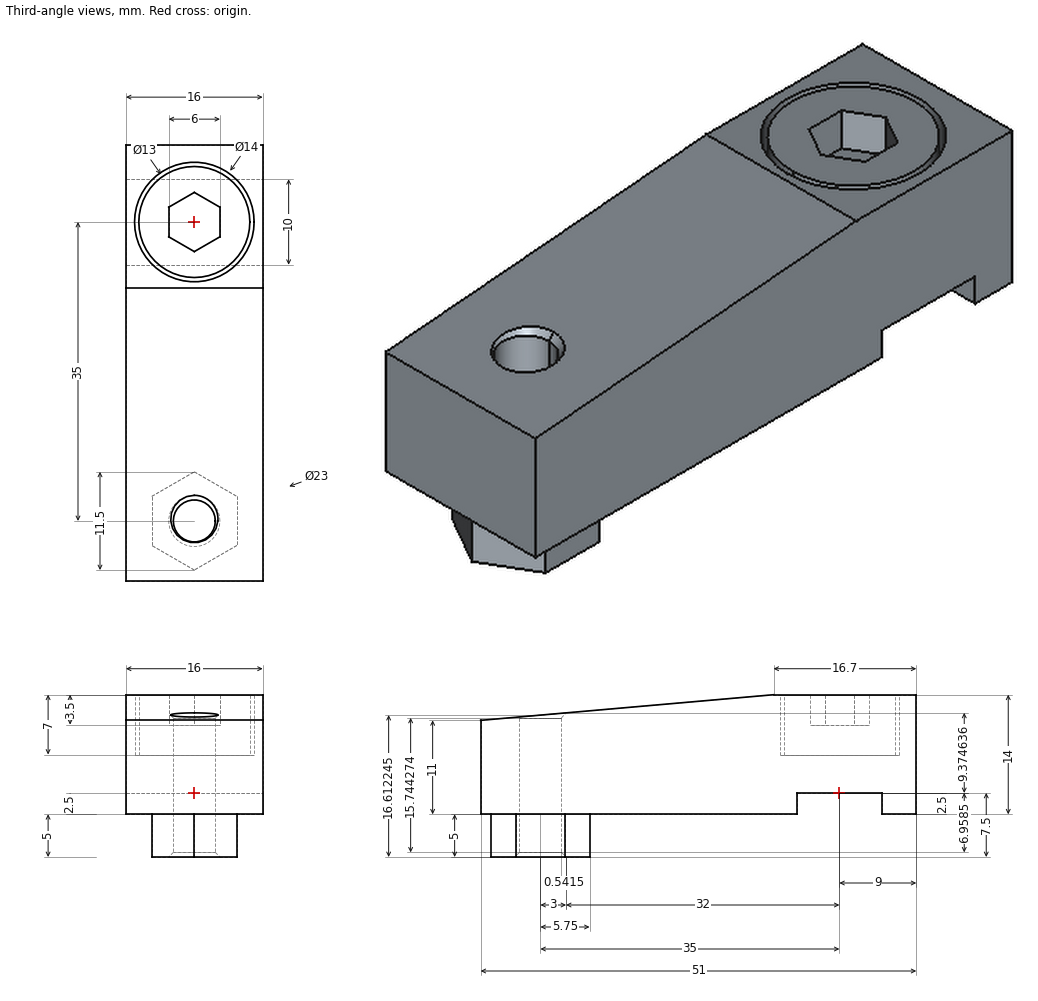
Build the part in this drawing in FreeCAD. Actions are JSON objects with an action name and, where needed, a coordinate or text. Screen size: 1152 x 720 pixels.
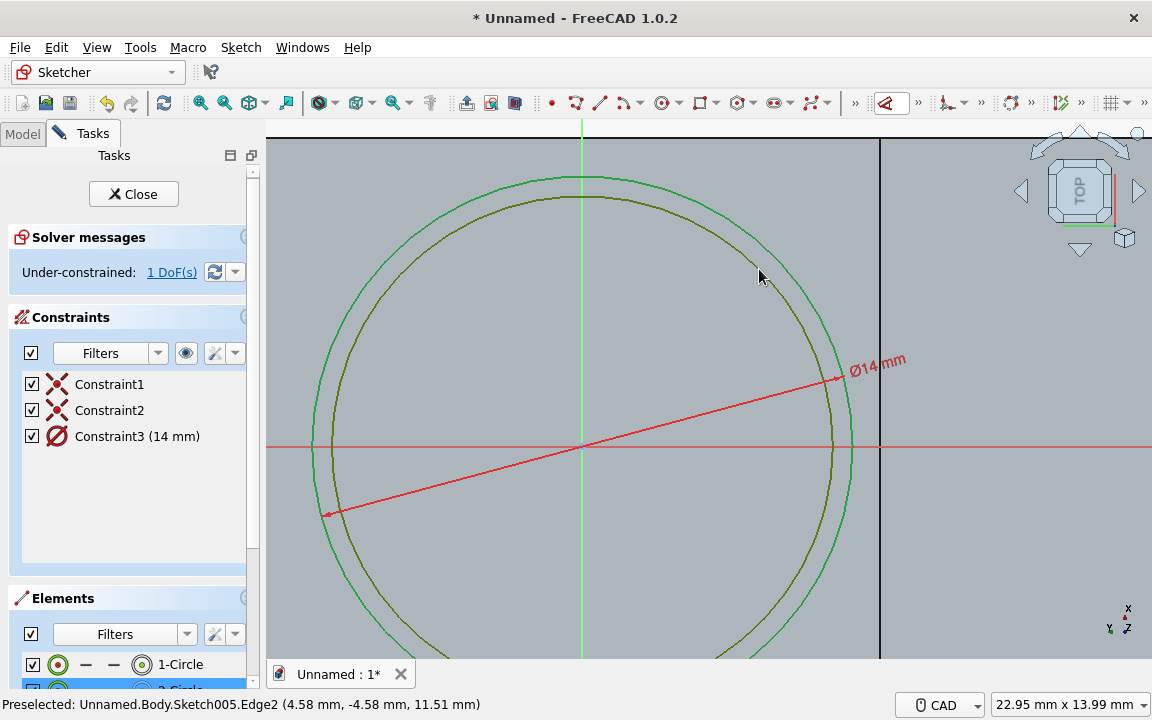
{"action": "key", "text": "k o"}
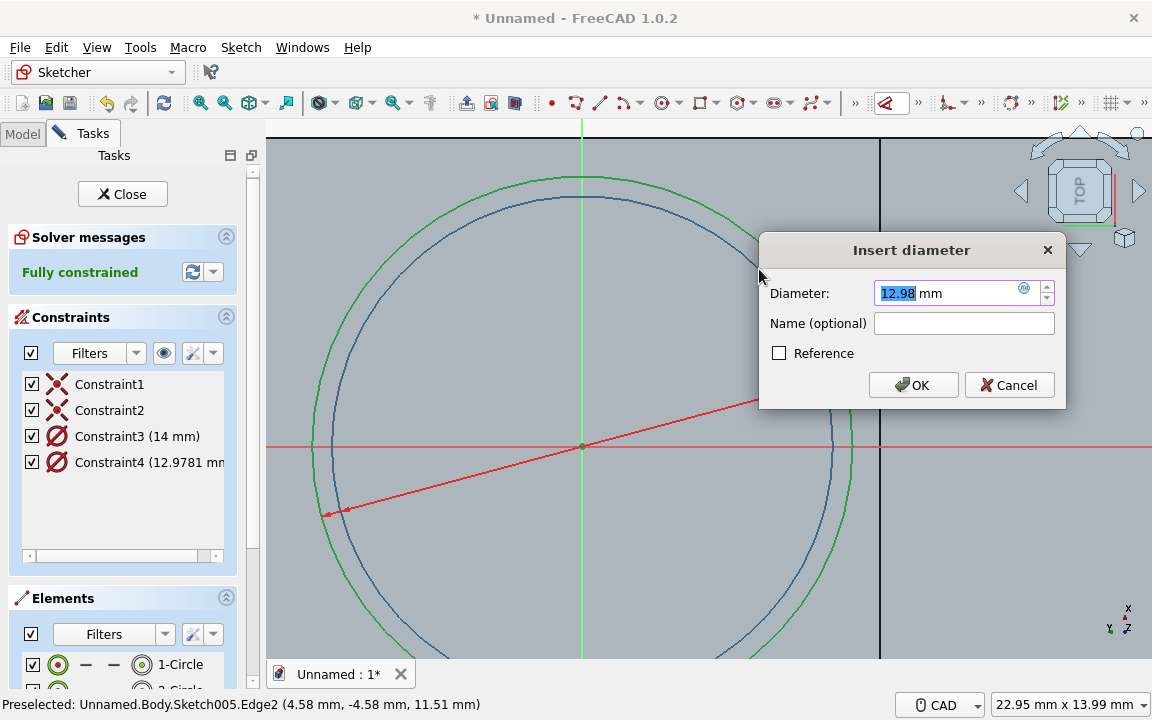
{"action": "type", "text": "13"}
{"action": "key", "text": "Return"}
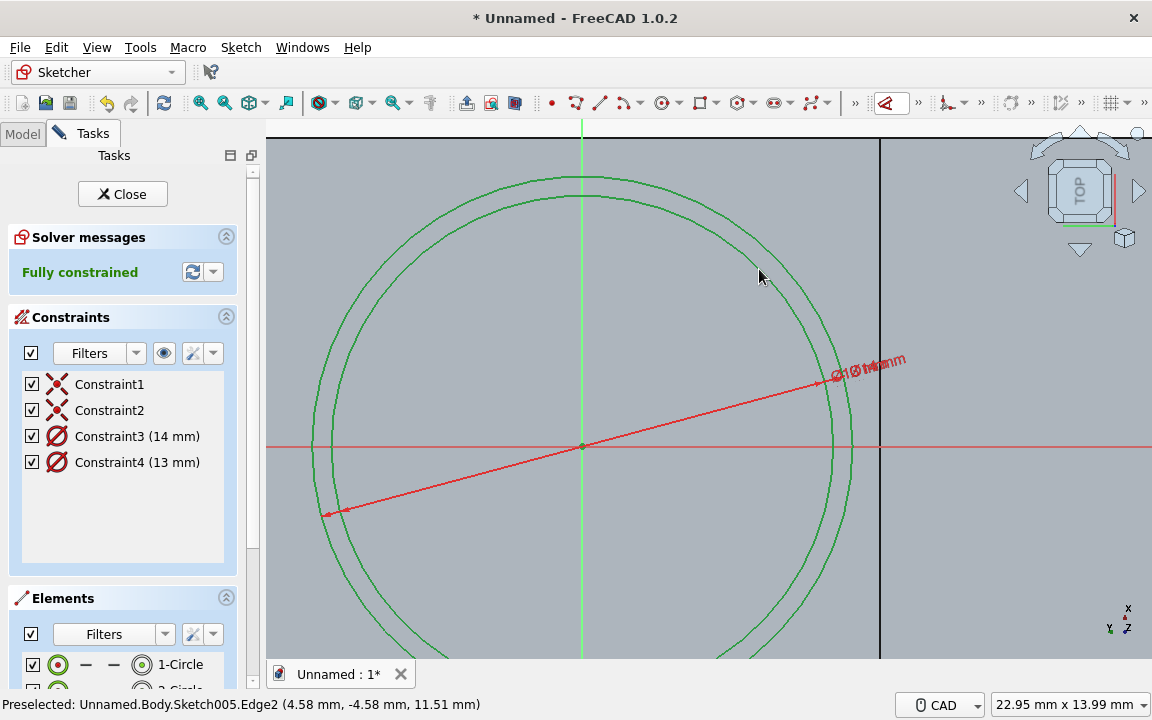
{"action": "left_click", "coordinate": [123, 194]}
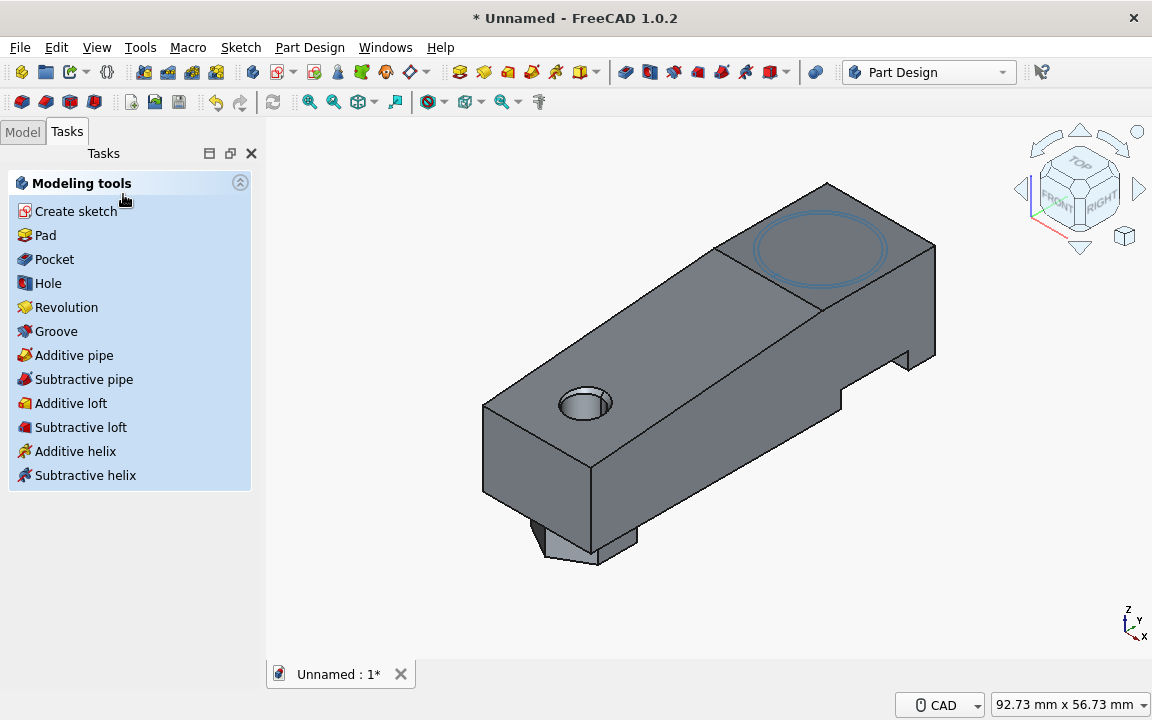
{"action": "left_click", "coordinate": [626, 72]}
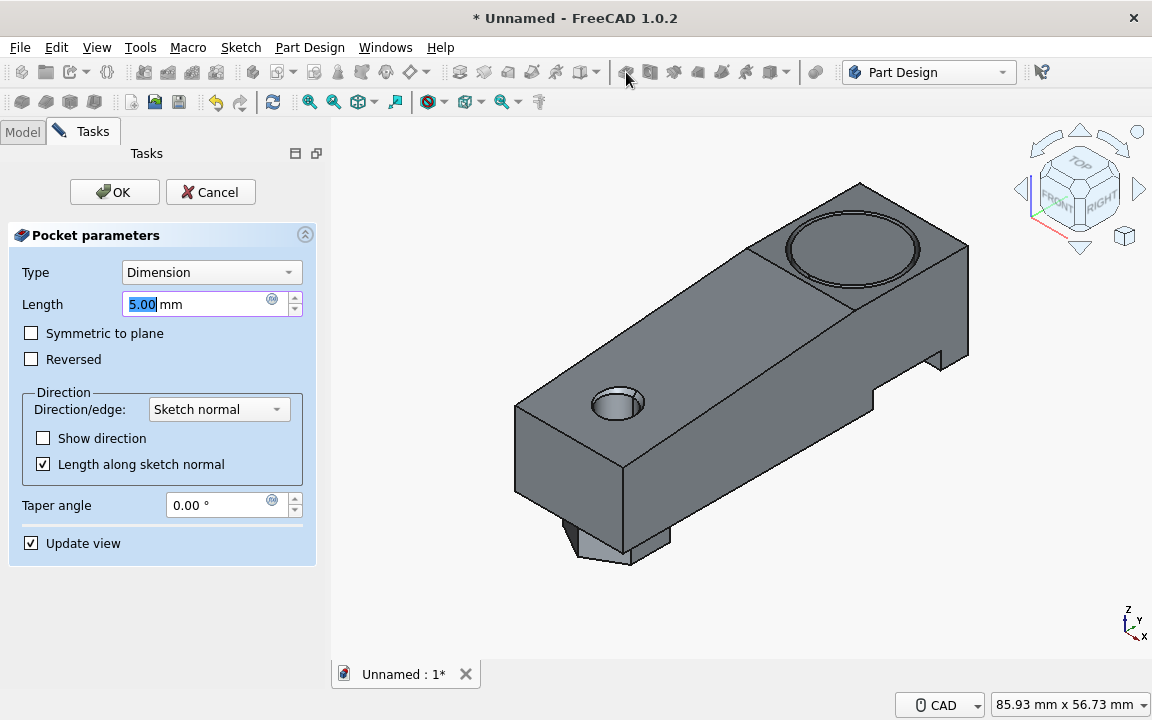
{"action": "type", "text": "7"}
{"action": "key", "text": "Tab"}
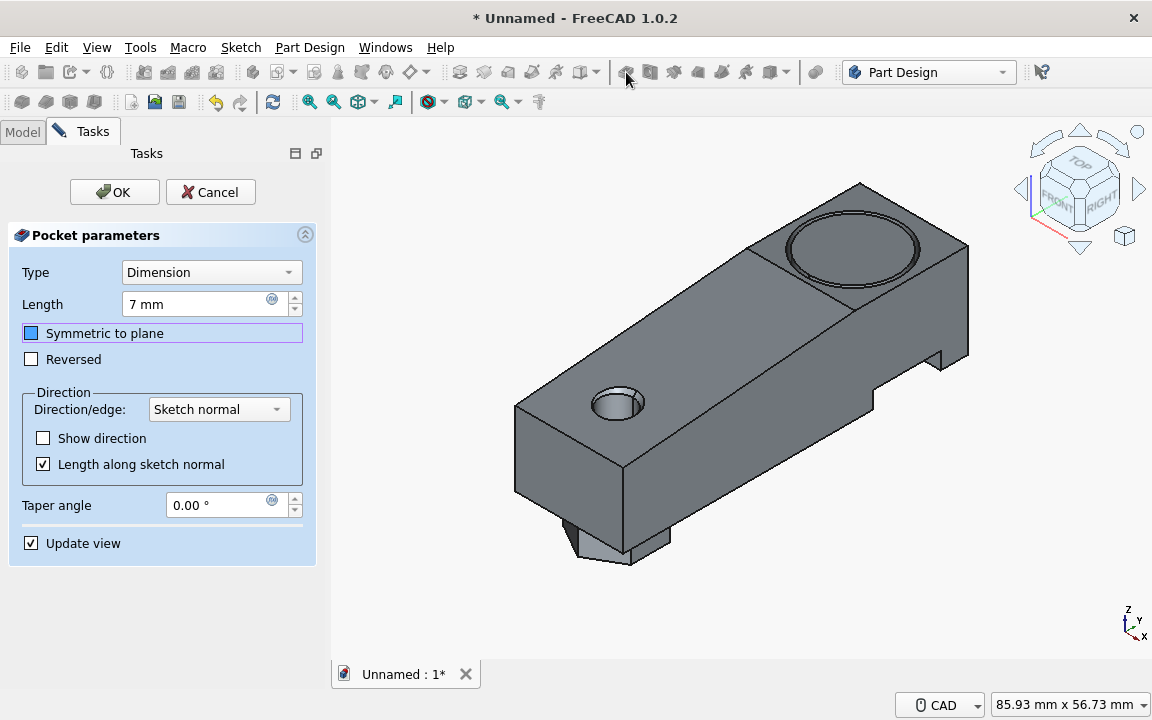
{"action": "left_click", "coordinate": [115, 192]}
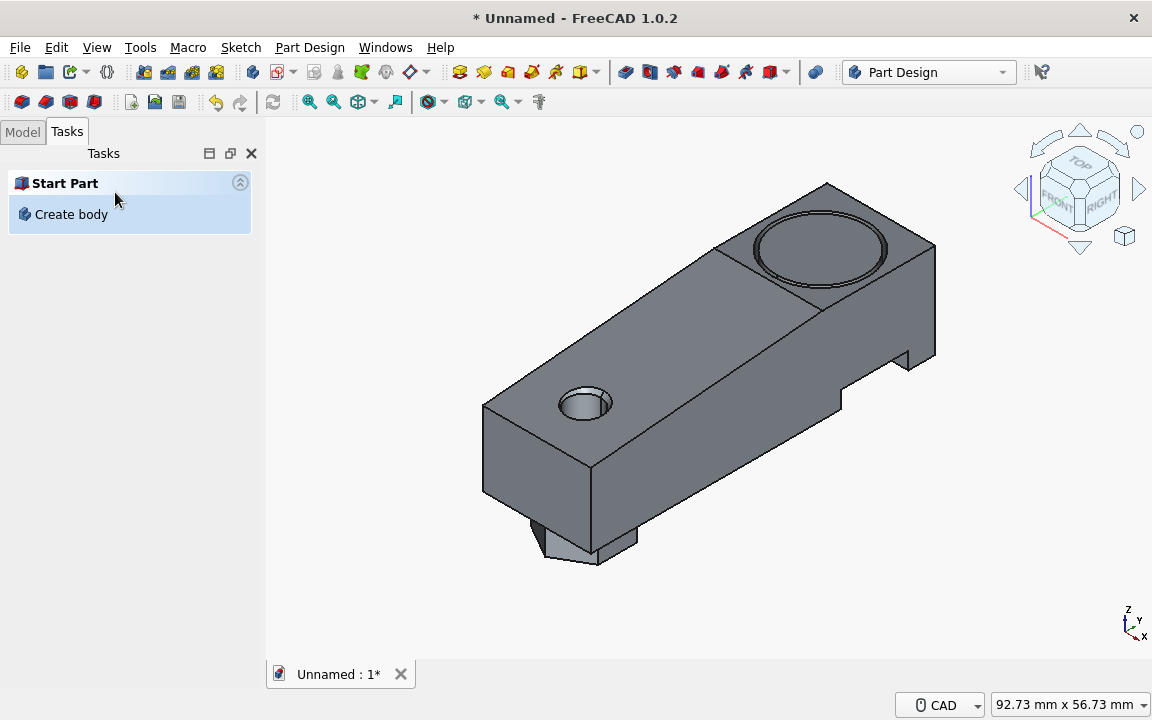
{"action": "left_click", "coordinate": [820, 249]}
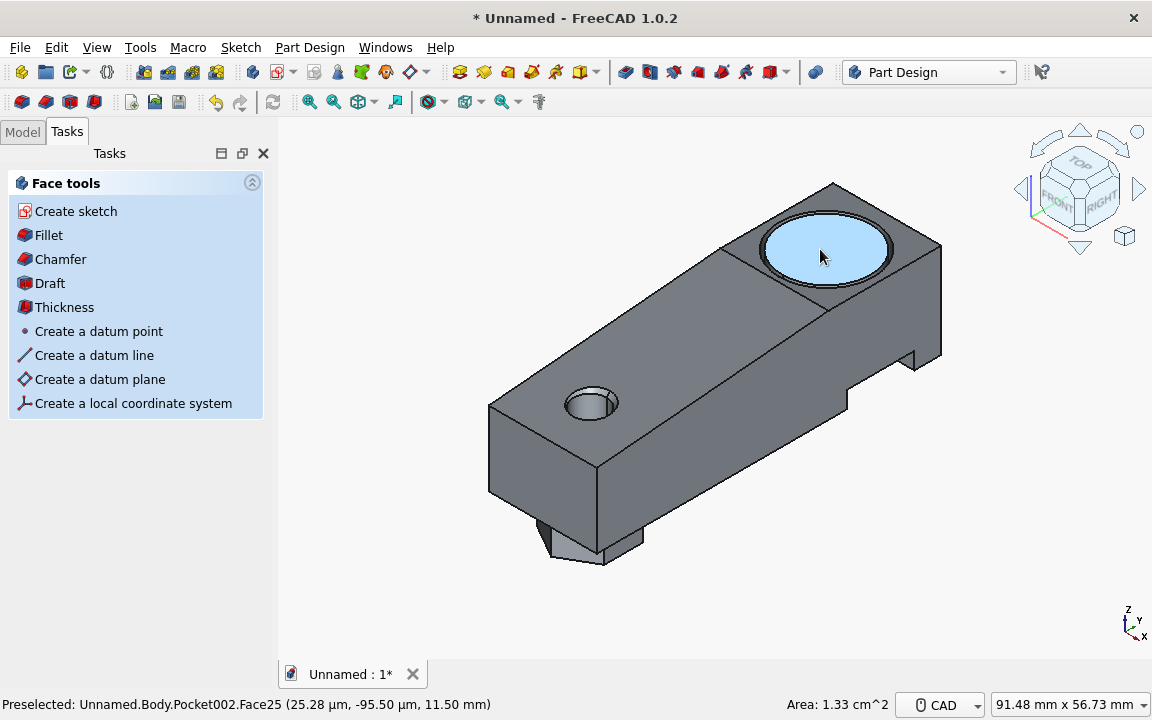
{"action": "left_click", "coordinate": [278, 72]}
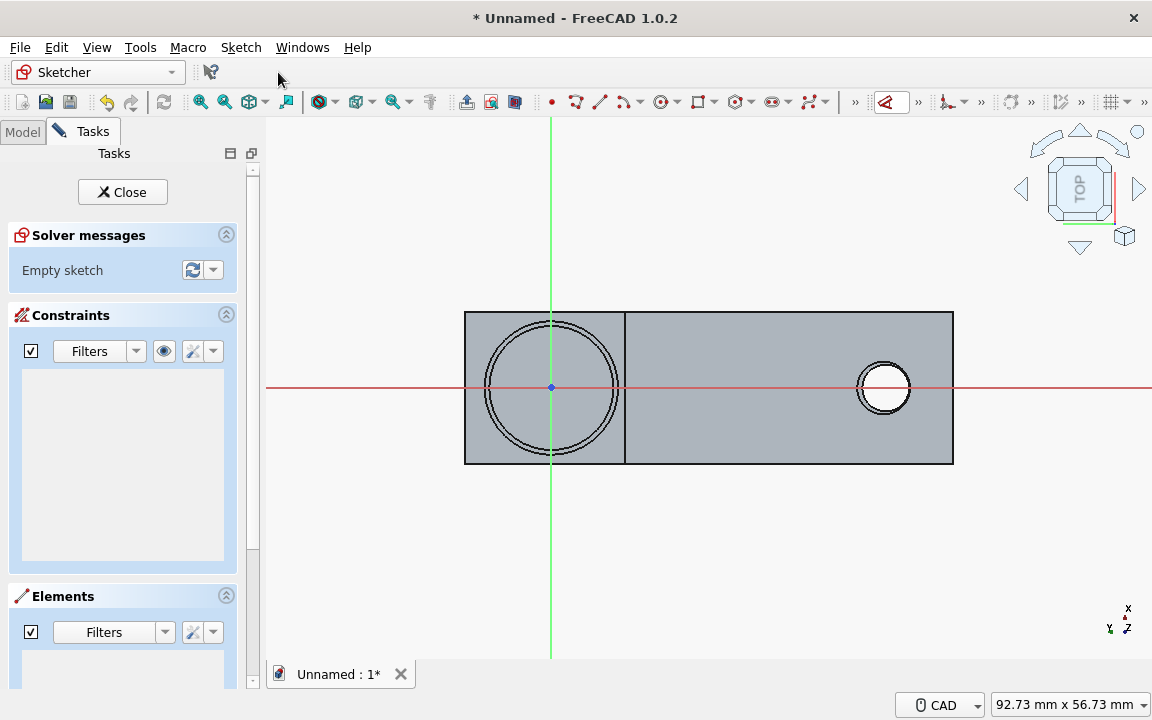
{"action": "scroll", "coordinate": [534, 388], "scroll_direction": "up", "scroll_amount": 9}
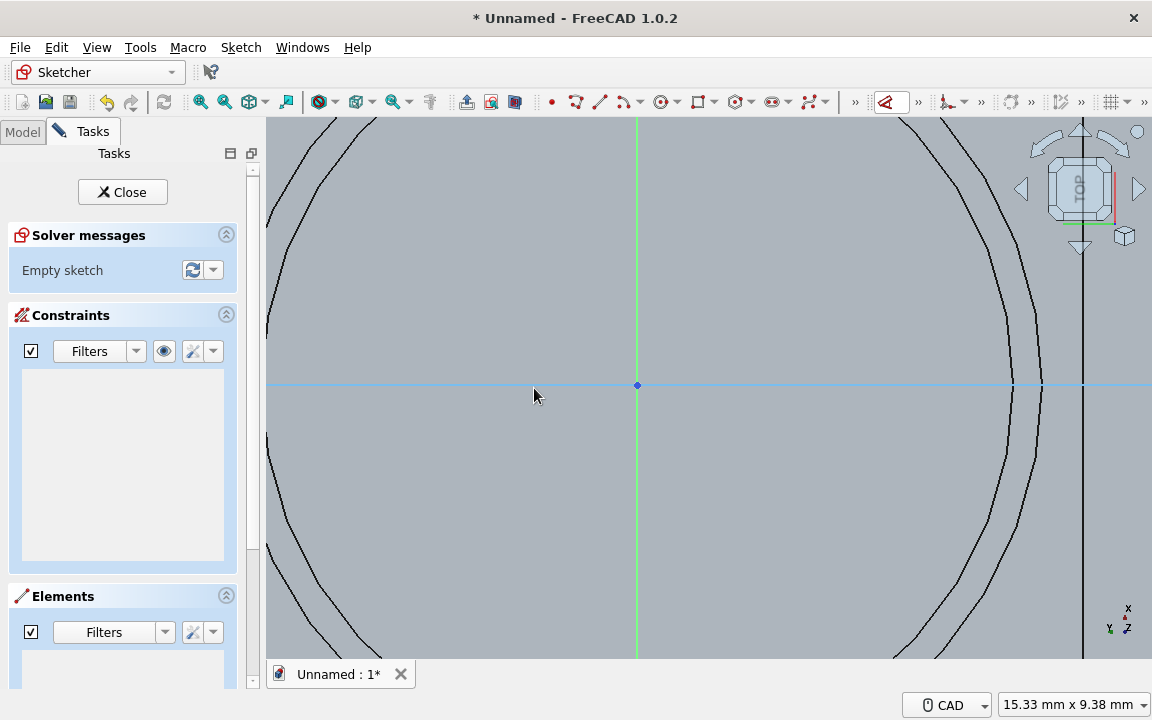
{"action": "key", "text": "g p 6"}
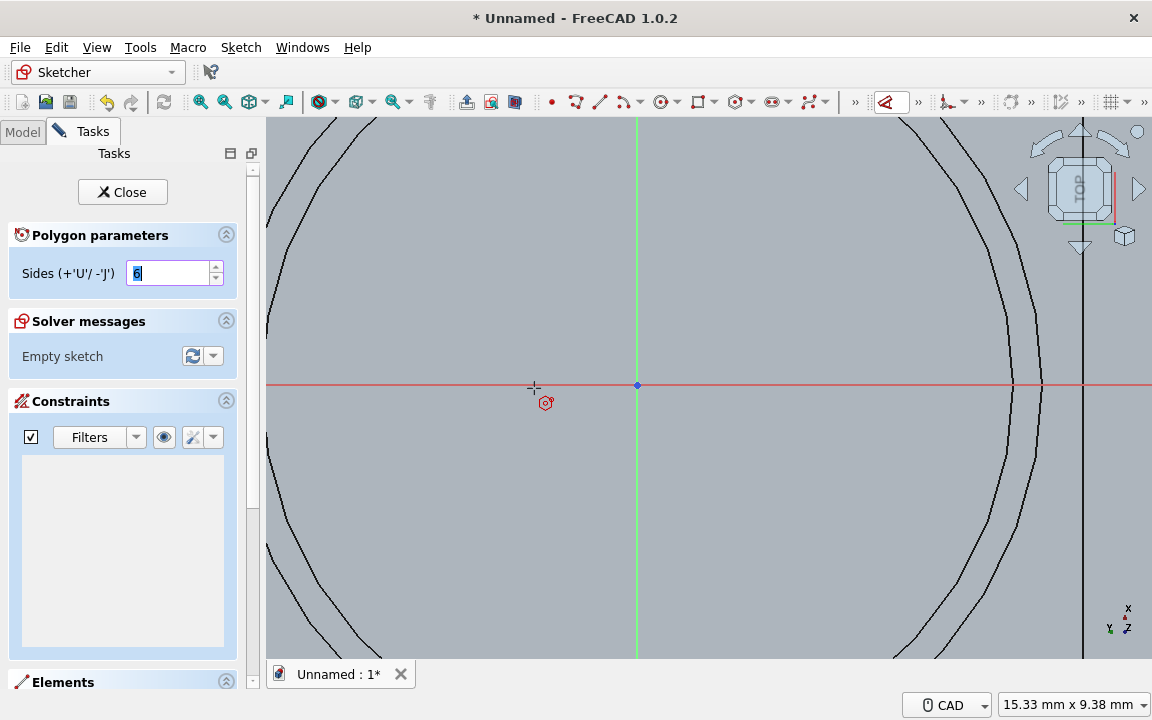
{"action": "left_click", "coordinate": [637, 385]}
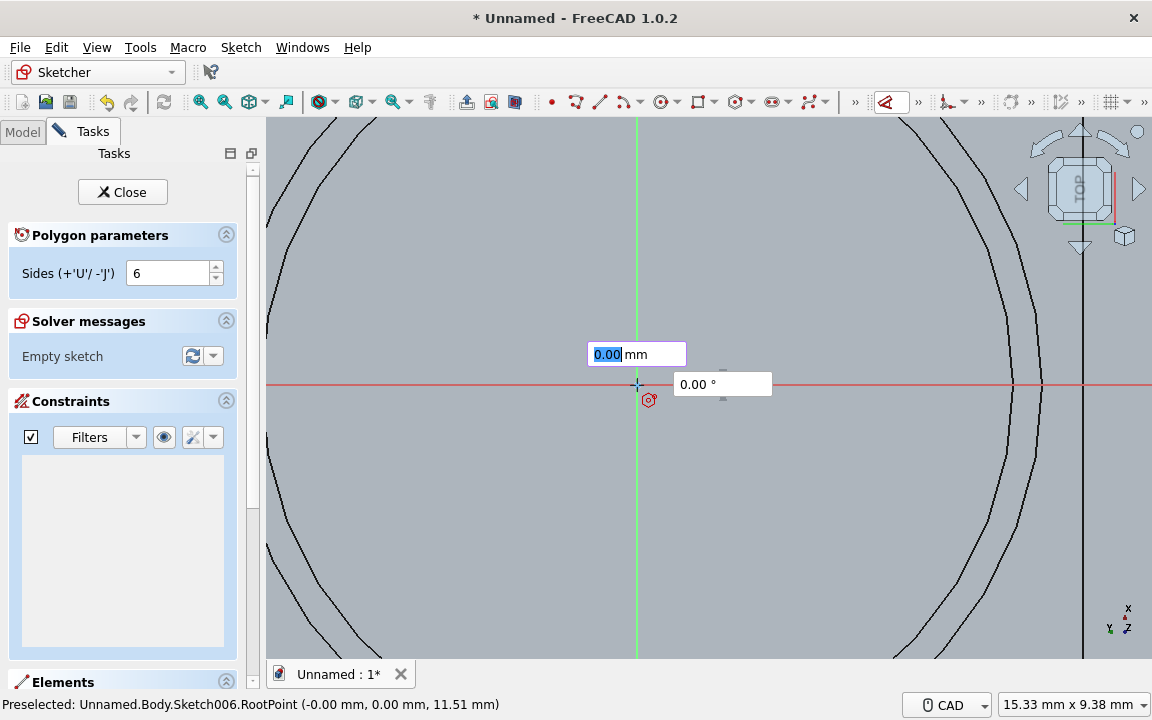
{"action": "left_click", "coordinate": [838, 385]}
{"action": "right_click", "coordinate": [838, 385]}